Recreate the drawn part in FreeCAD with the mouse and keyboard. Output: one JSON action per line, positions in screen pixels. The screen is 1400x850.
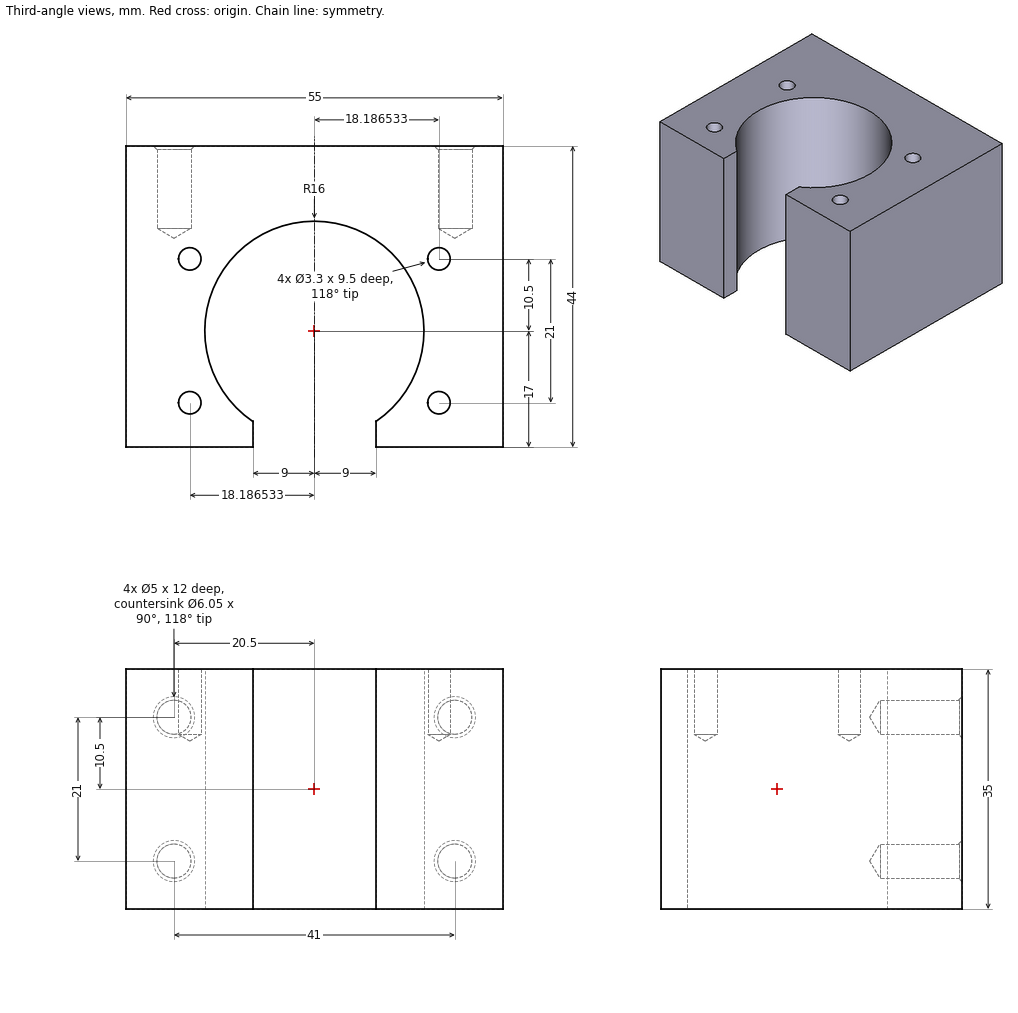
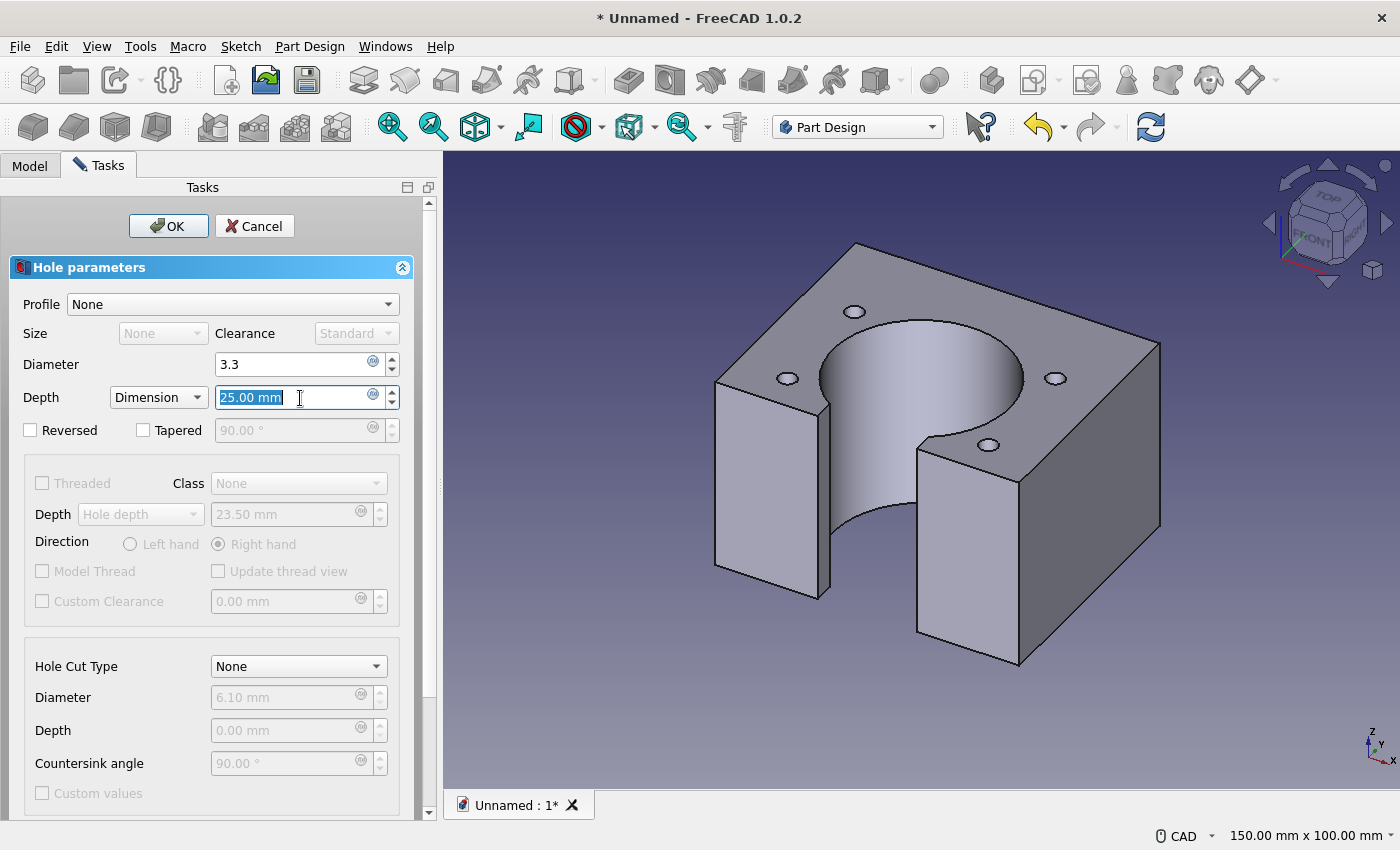
{"action": "type", "text": "9.5"}
{"action": "key", "text": "Tab"}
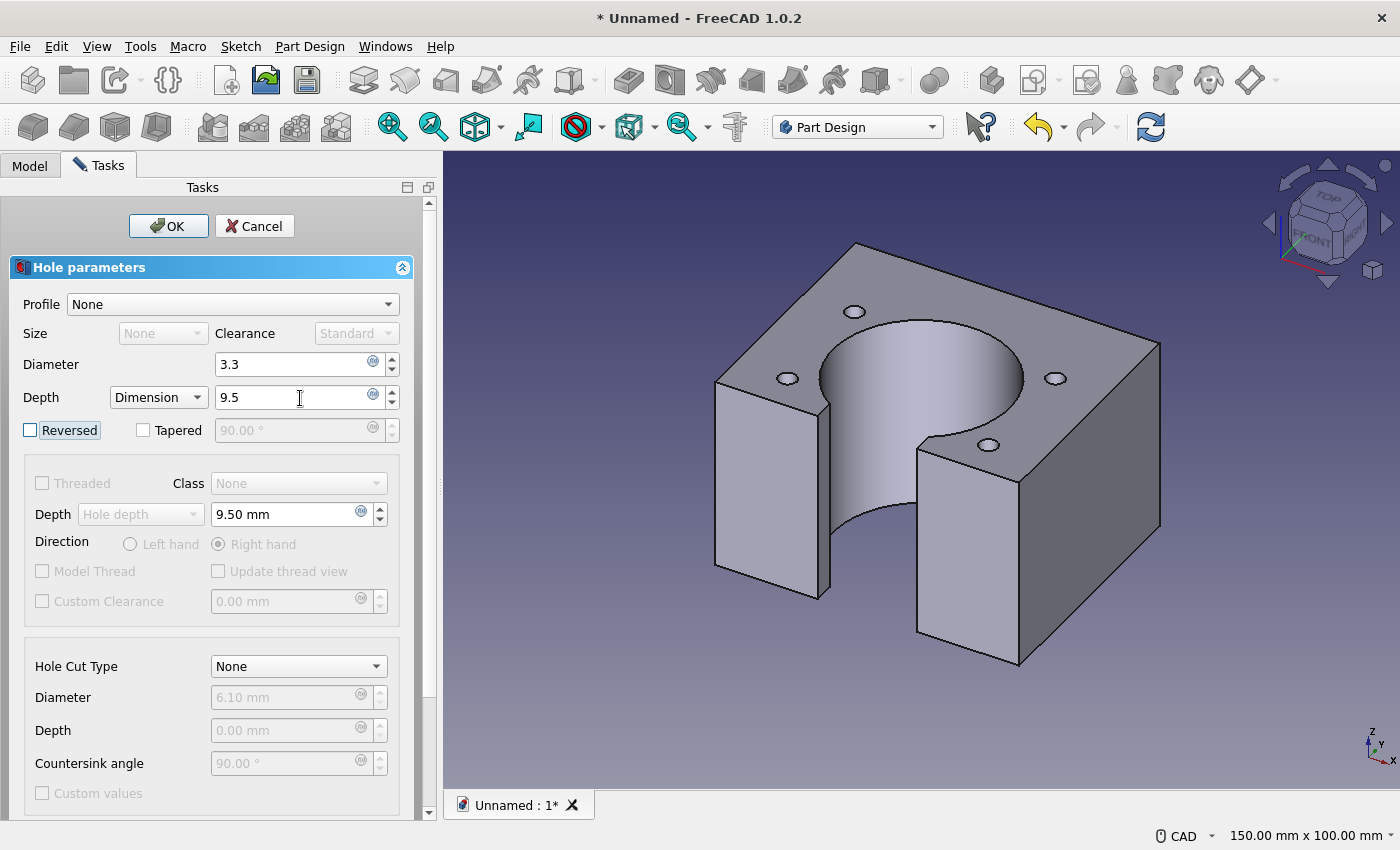
{"action": "left_click", "coordinate": [169, 226]}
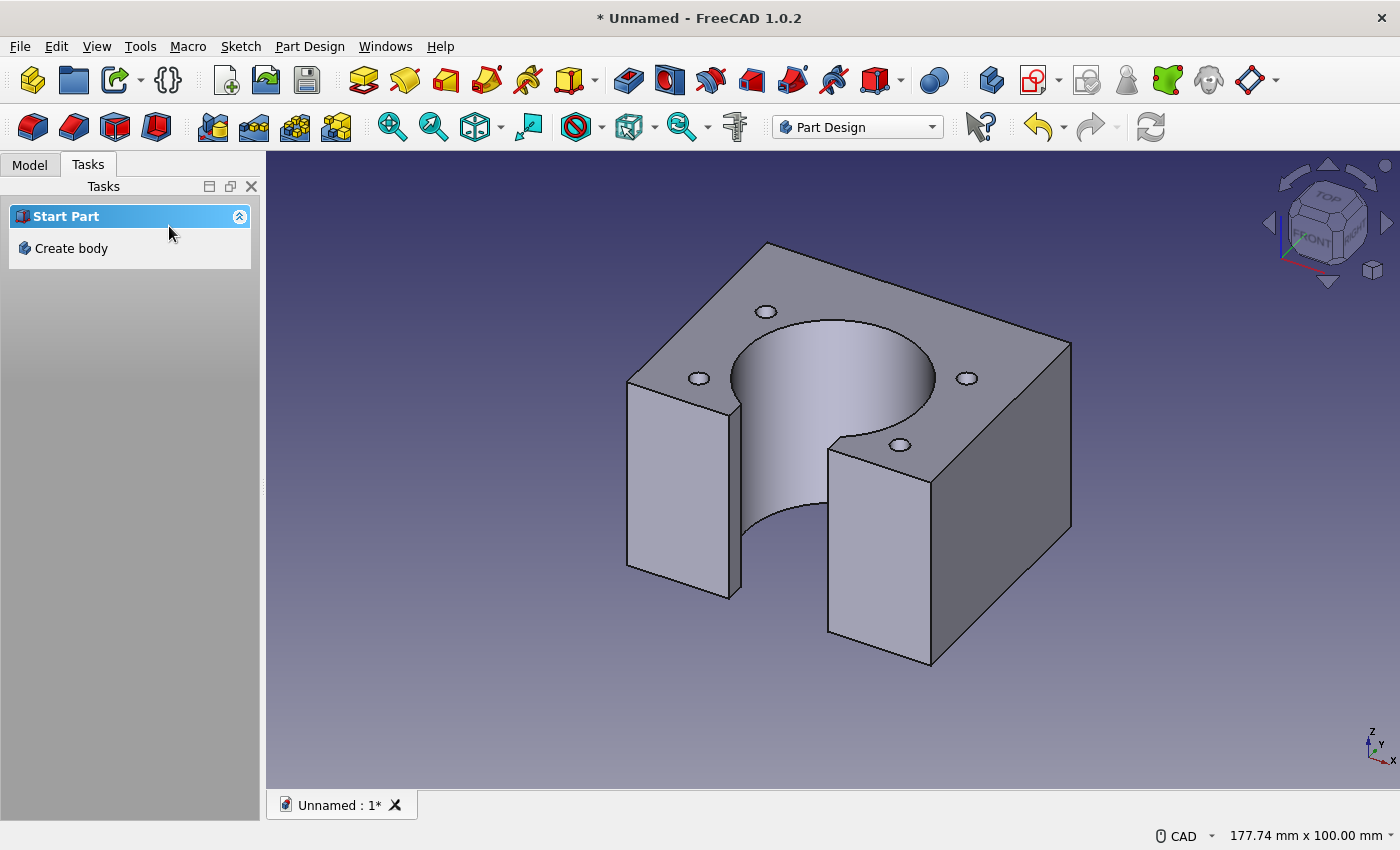
{"action": "key", "text": "4"}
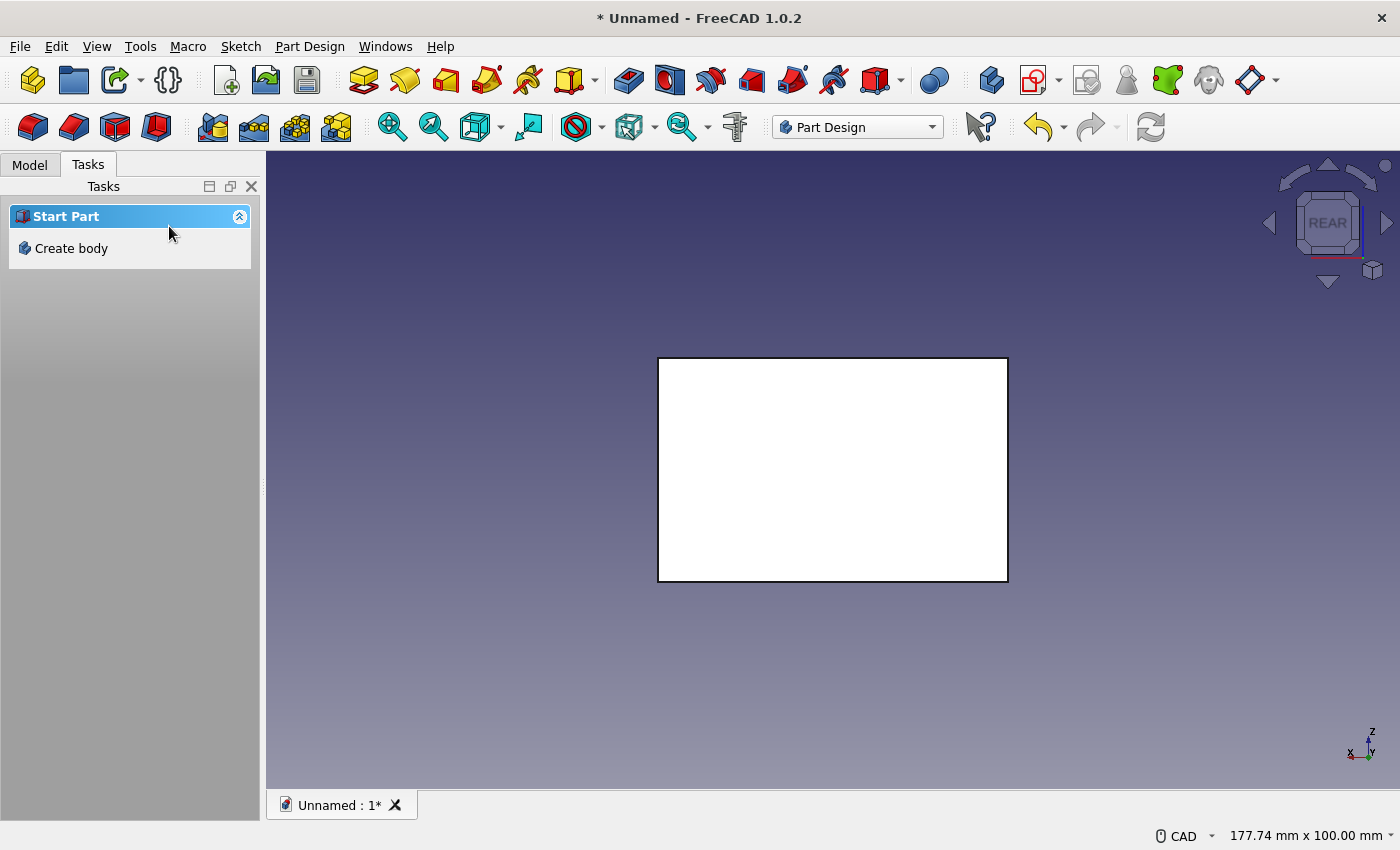
{"action": "left_click", "coordinate": [393, 128]}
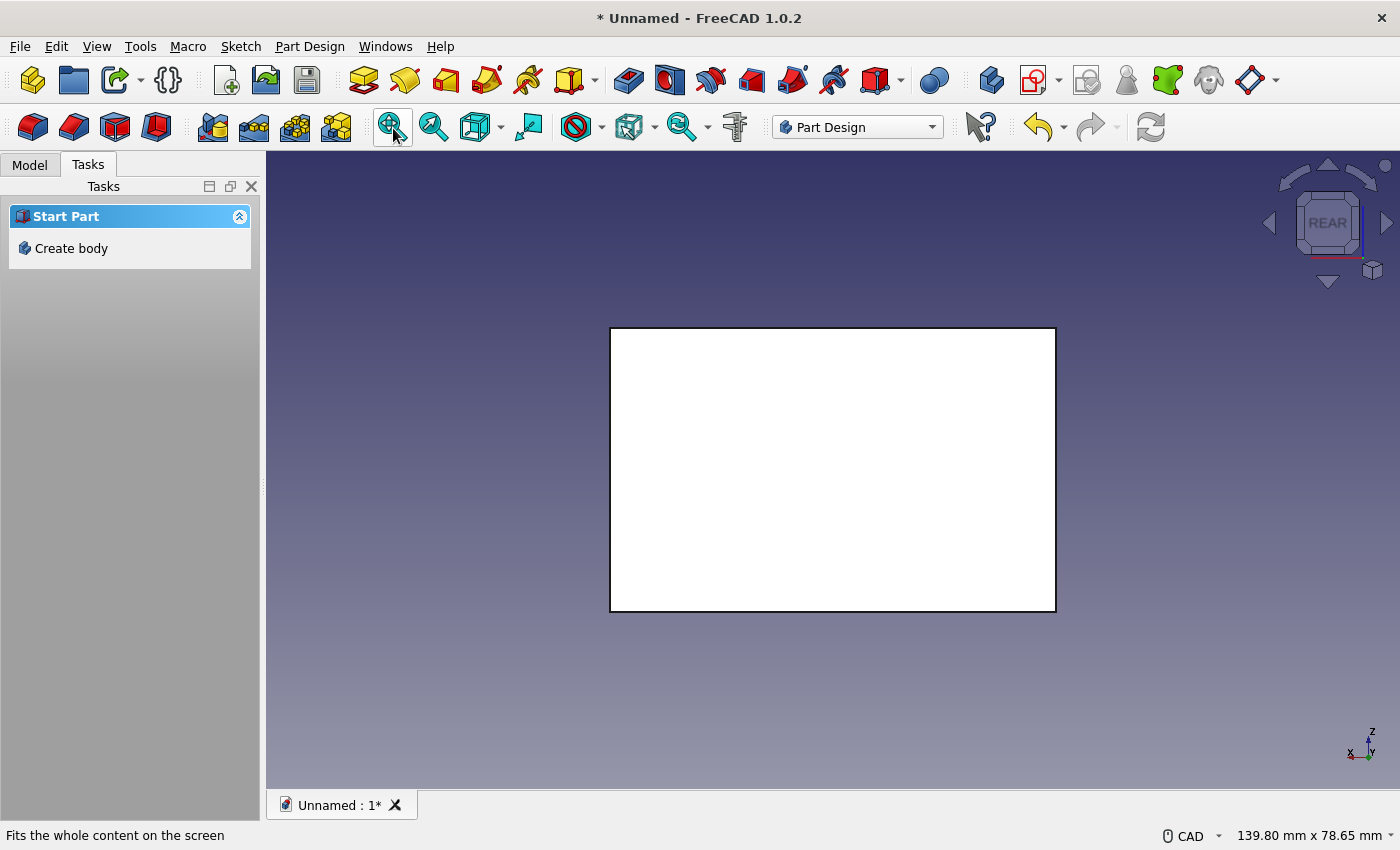
{"action": "left_click", "coordinate": [769, 469]}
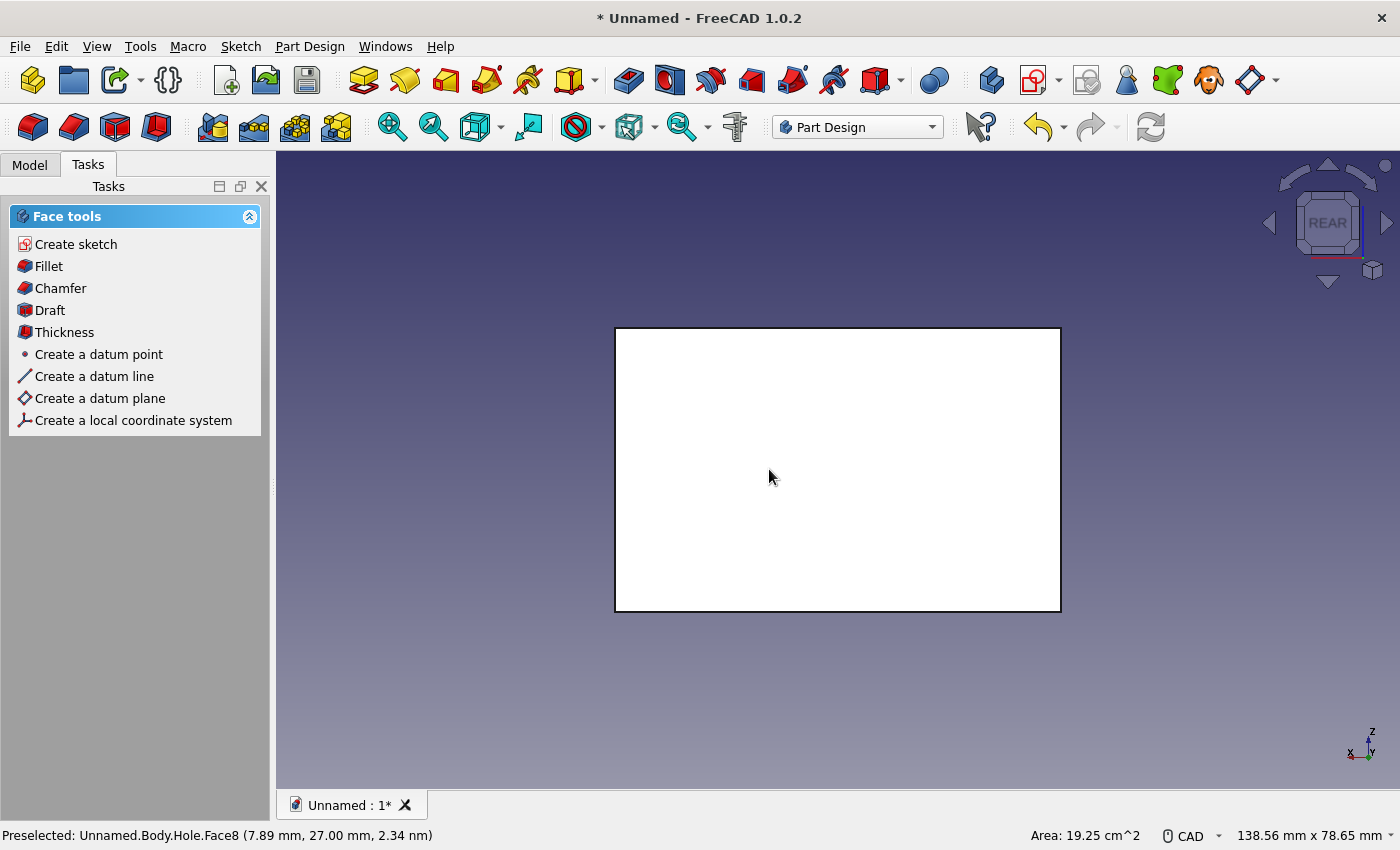
{"action": "left_click", "coordinate": [1032, 80]}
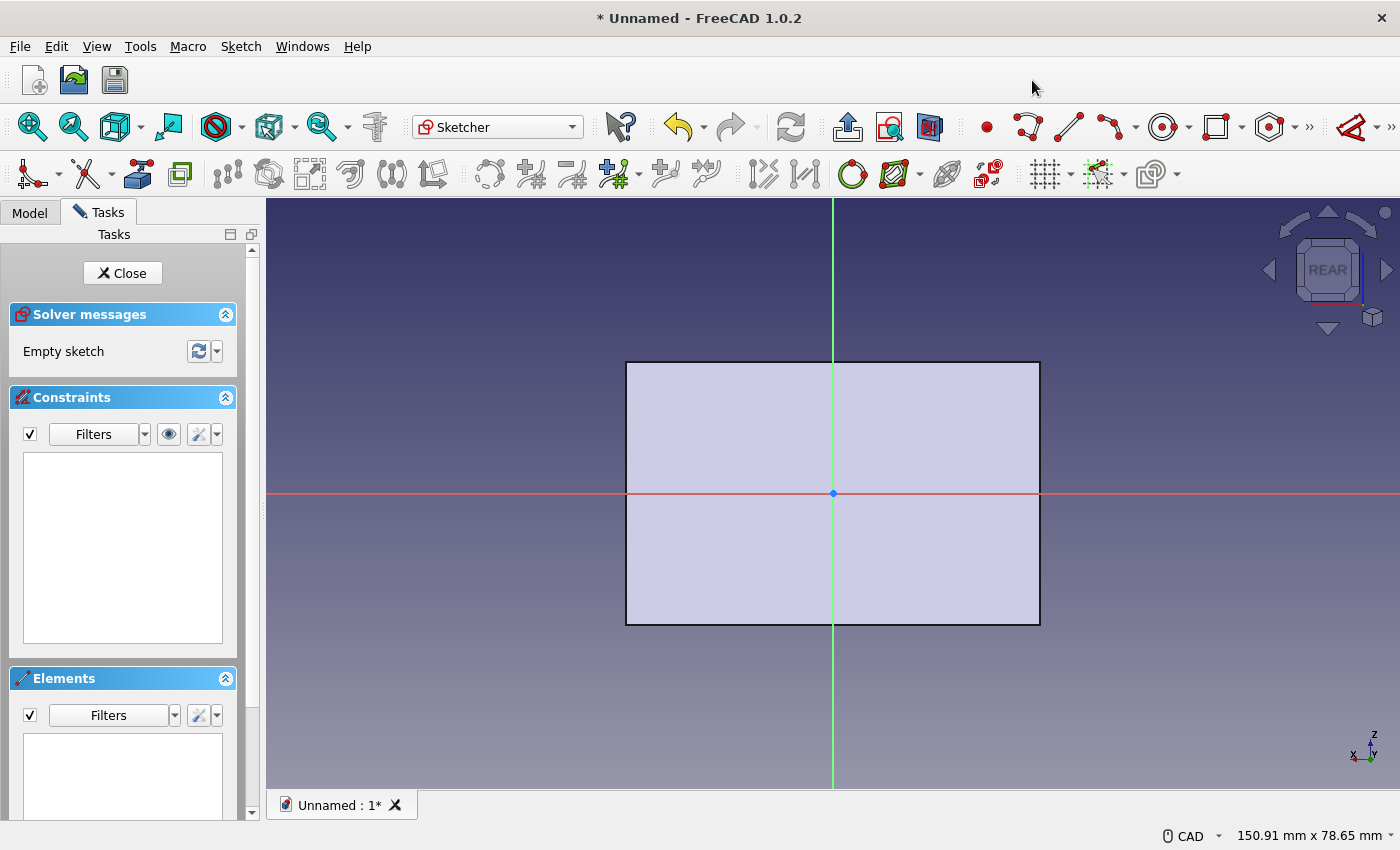
{"action": "scroll", "coordinate": [916, 494], "scroll_direction": "up", "scroll_amount": 3}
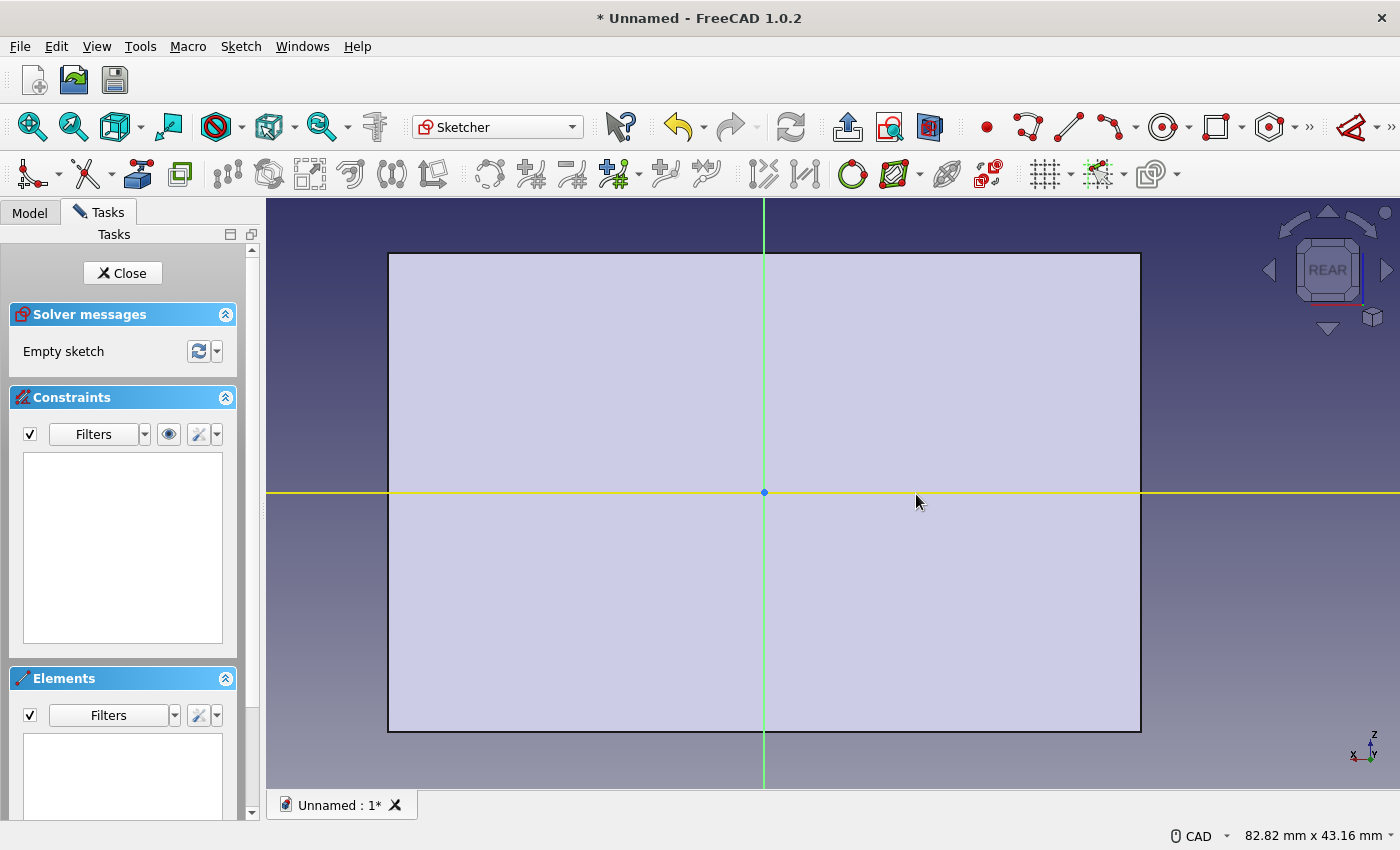
{"action": "left_click", "coordinate": [1162, 128]}